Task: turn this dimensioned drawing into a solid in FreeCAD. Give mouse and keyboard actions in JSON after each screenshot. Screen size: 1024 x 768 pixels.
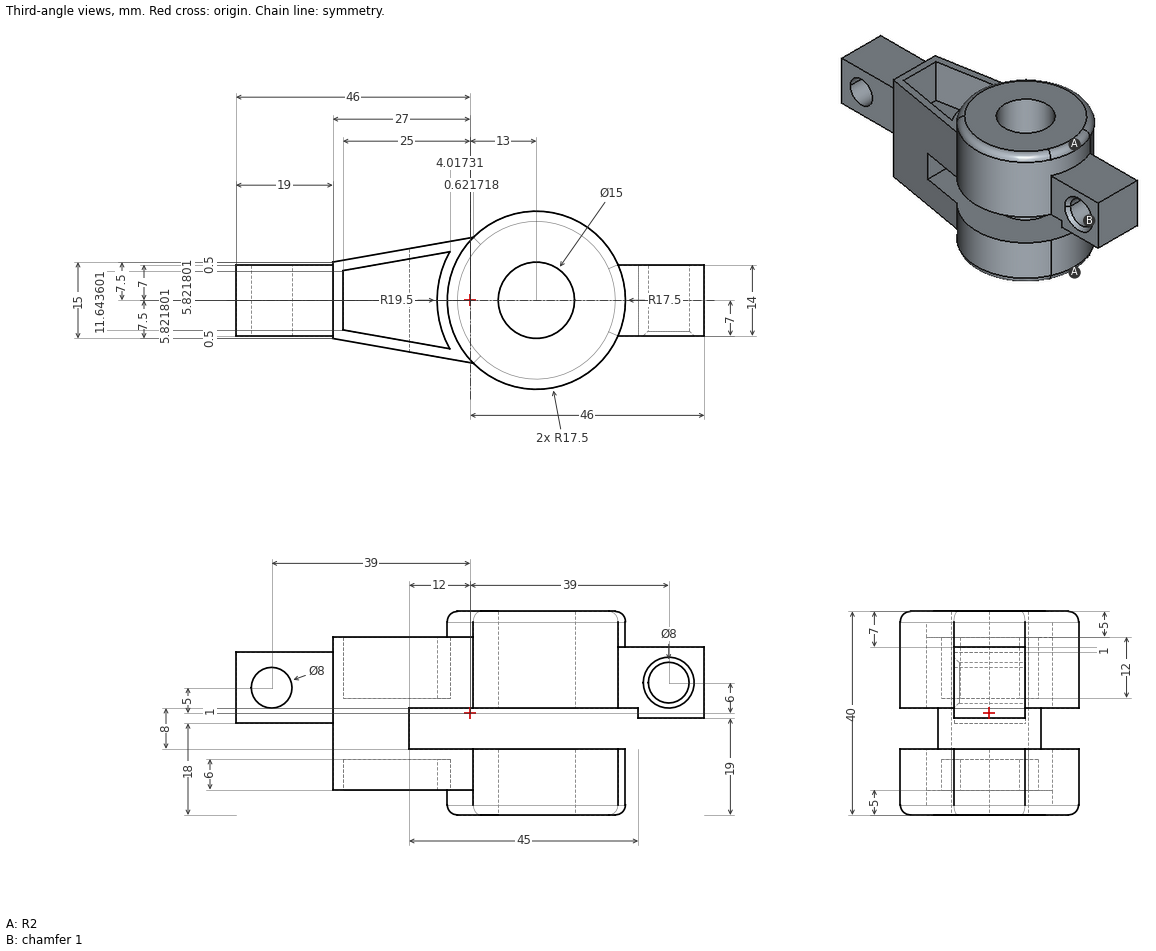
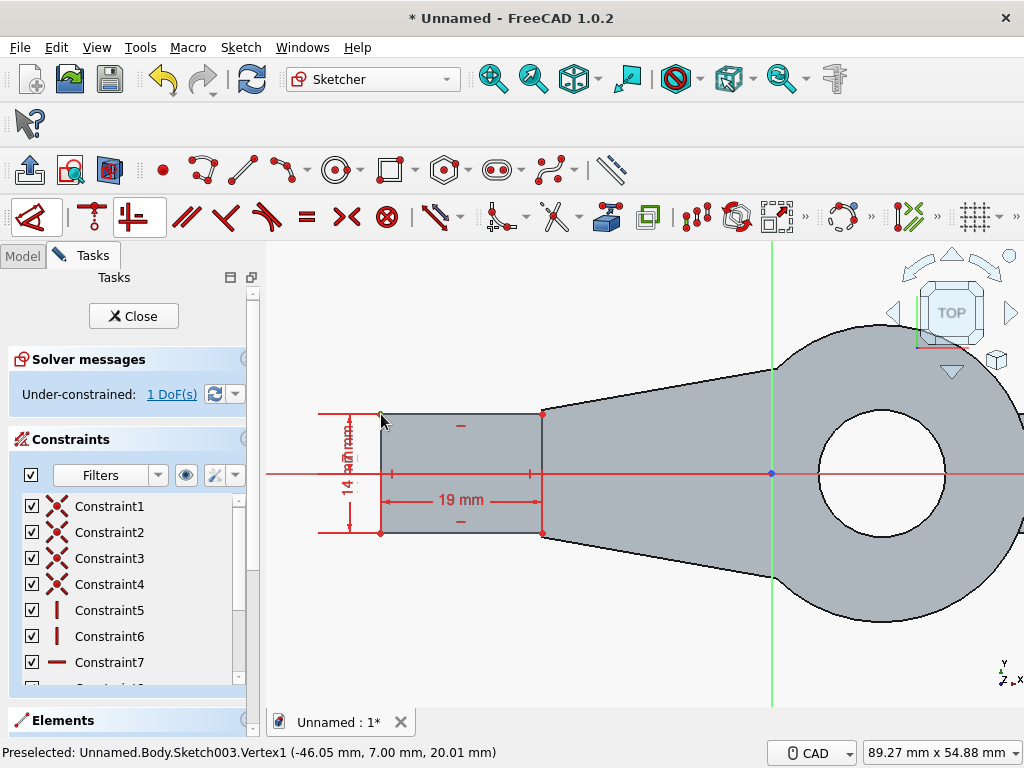
{"action": "key", "text": "l"}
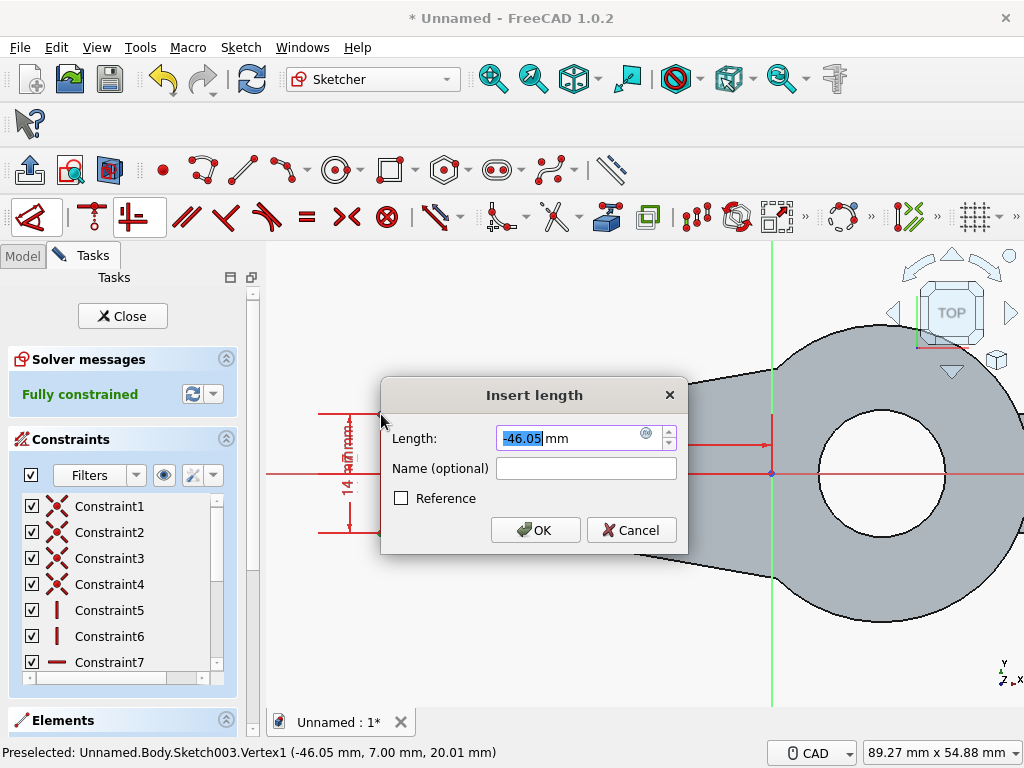
{"action": "type", "text": "-46"}
{"action": "key", "text": "Return"}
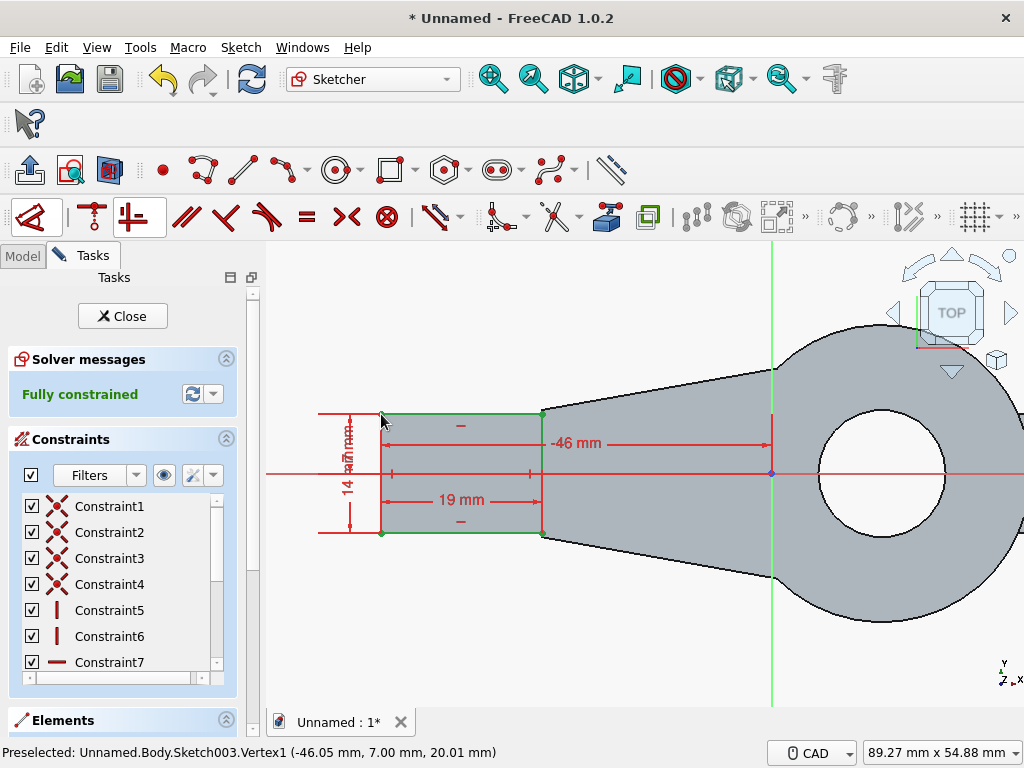
{"action": "left_click", "coordinate": [123, 316]}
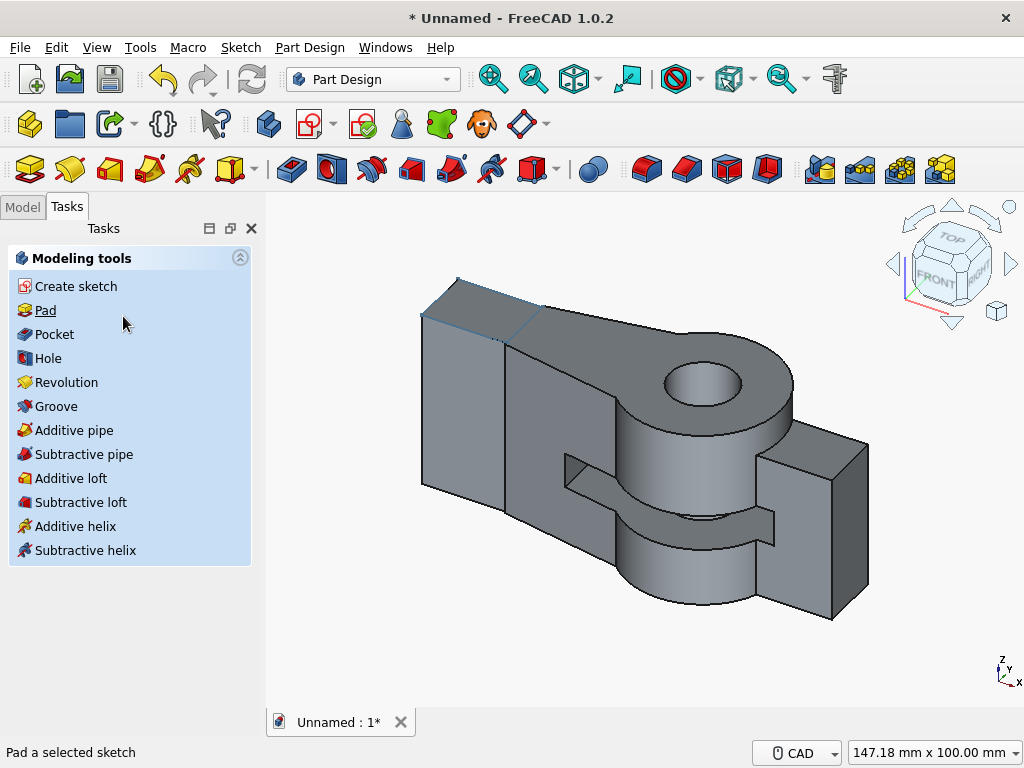
{"action": "left_click", "coordinate": [292, 170]}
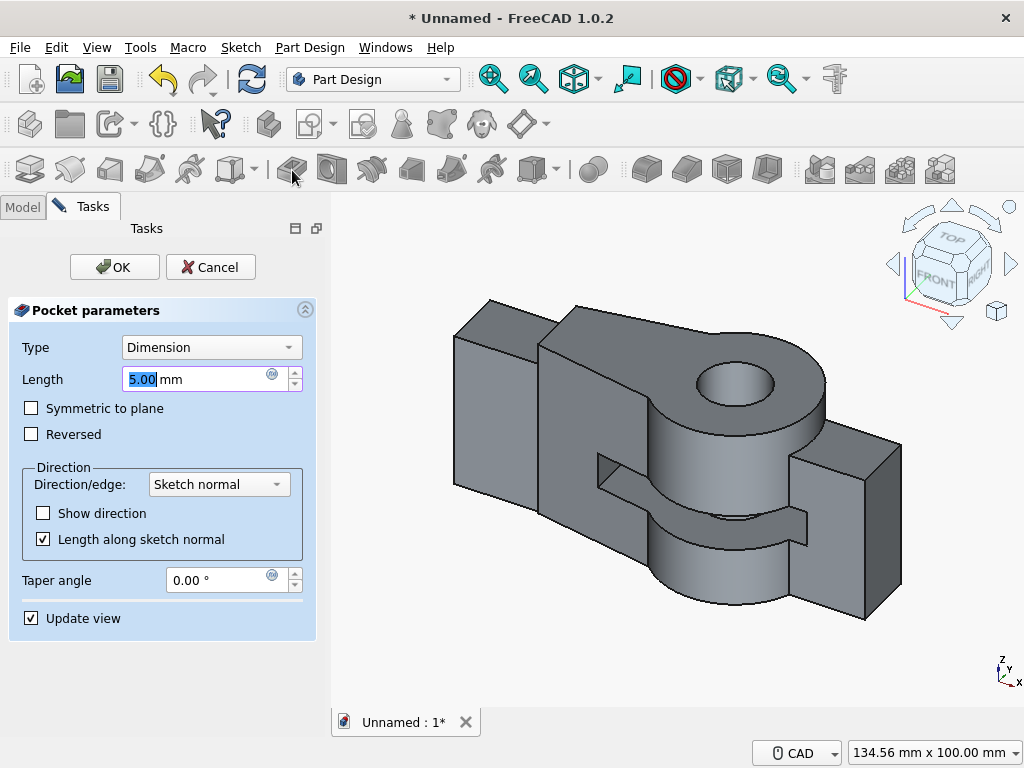
{"action": "type", "text": "7"}
{"action": "key", "text": "Tab"}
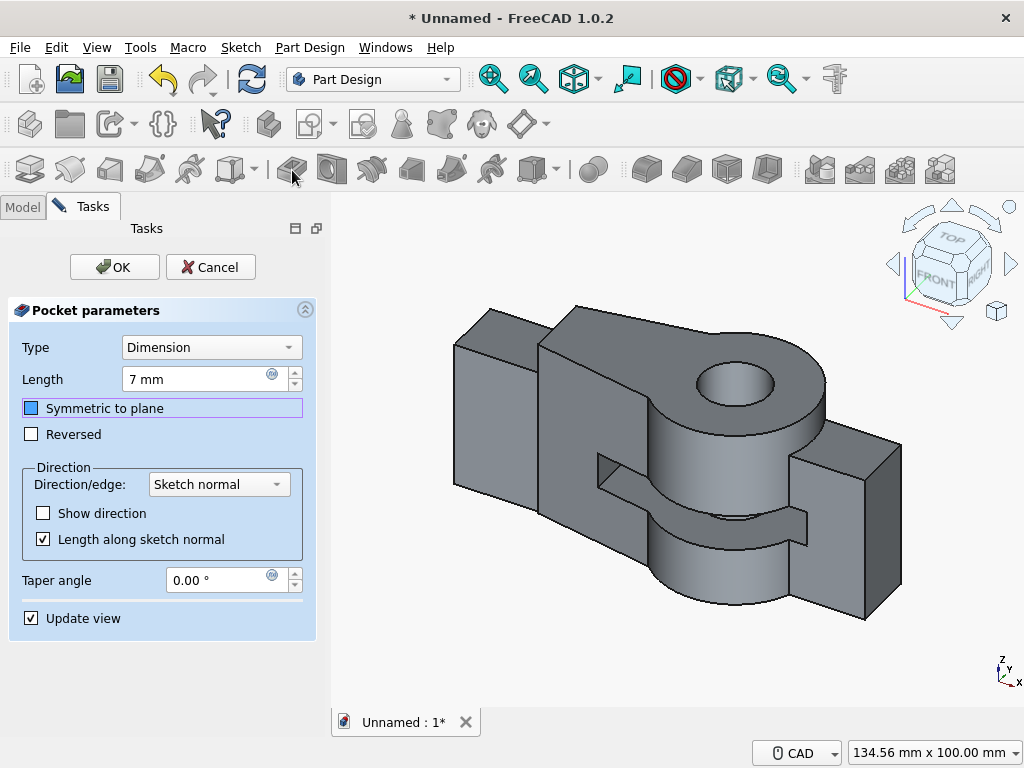
{"action": "left_click", "coordinate": [115, 267]}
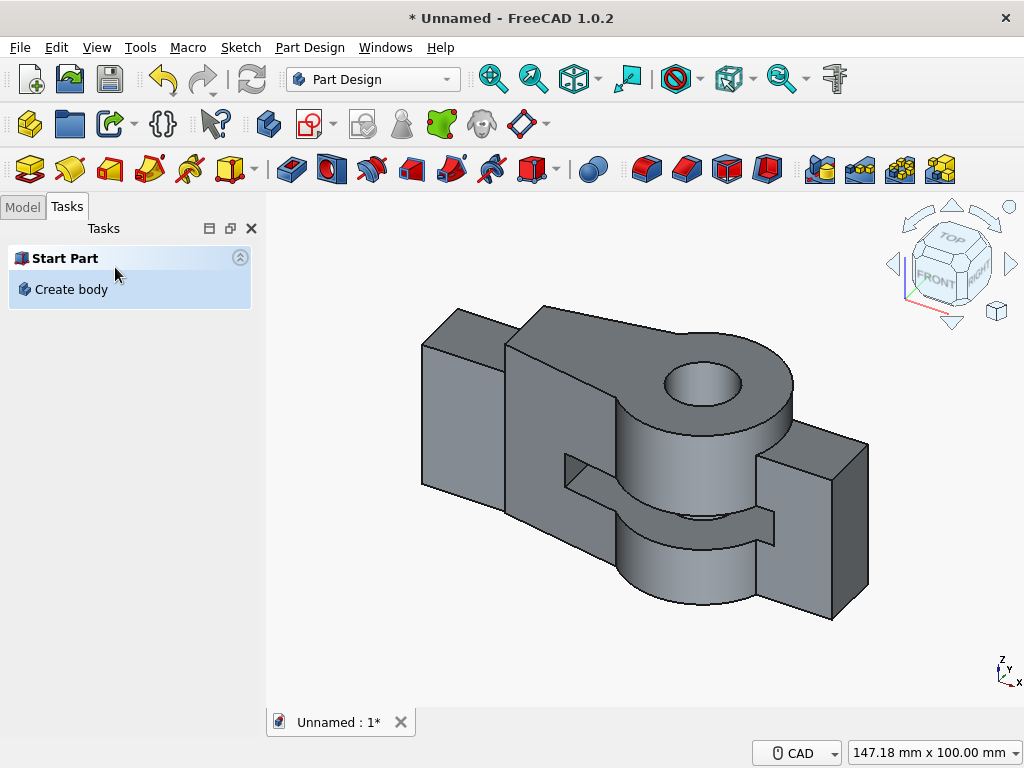
{"action": "left_click", "coordinate": [616, 355]}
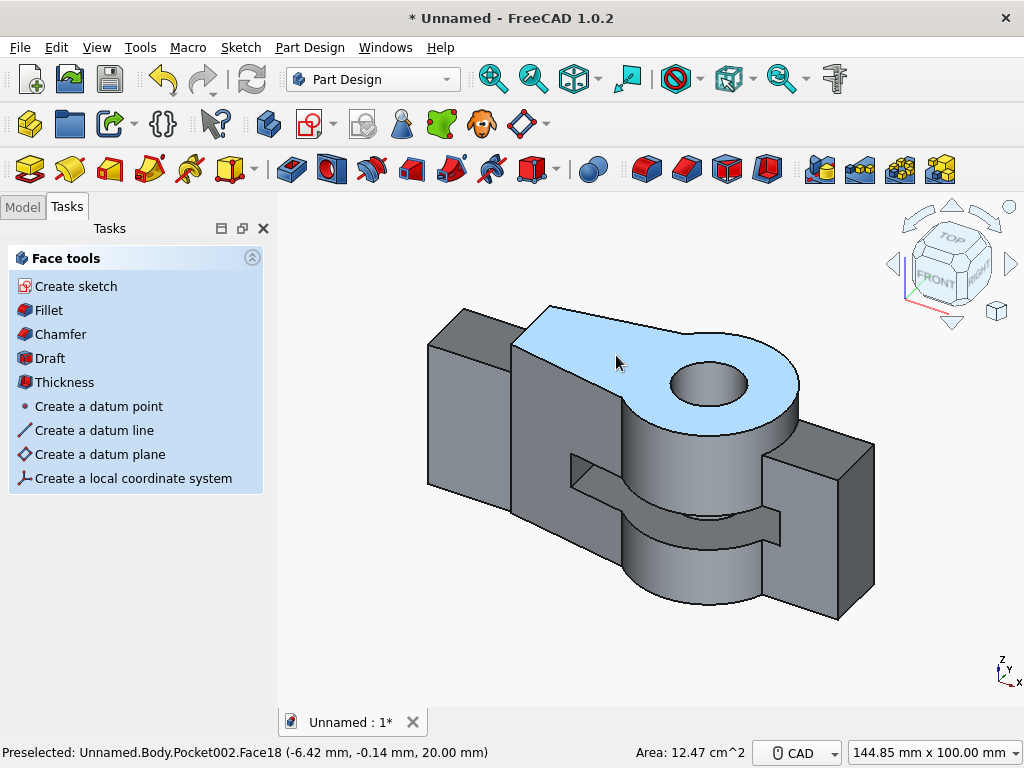
{"action": "left_click", "coordinate": [310, 124]}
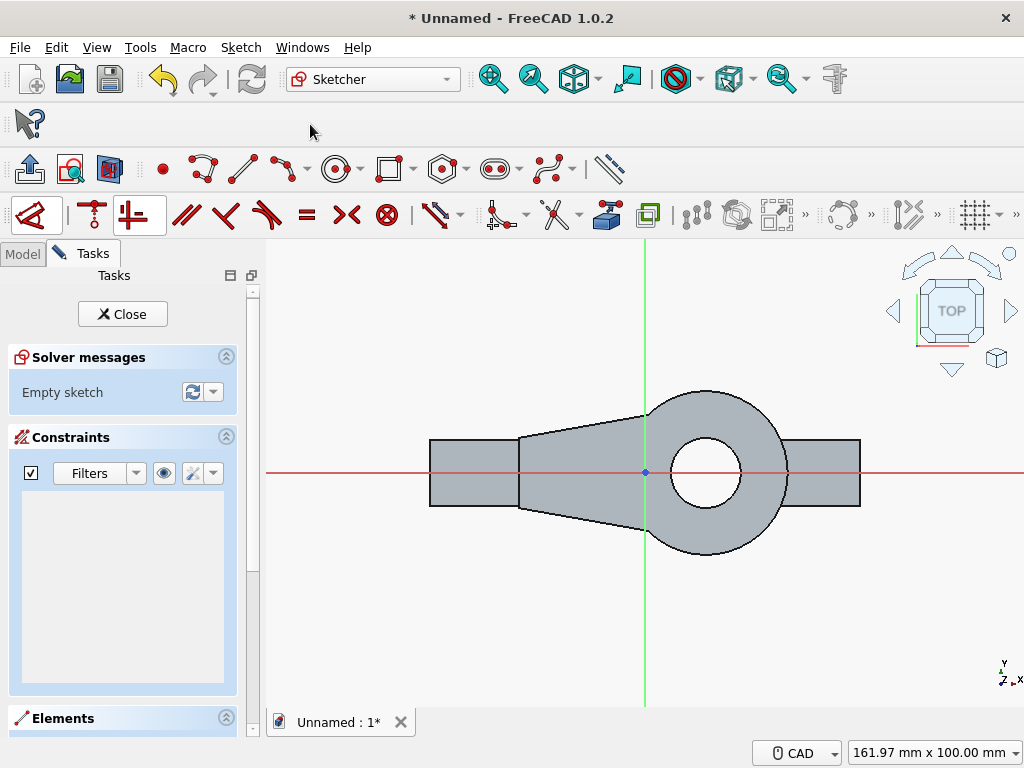
{"action": "scroll", "coordinate": [587, 473], "scroll_direction": "up", "scroll_amount": 5}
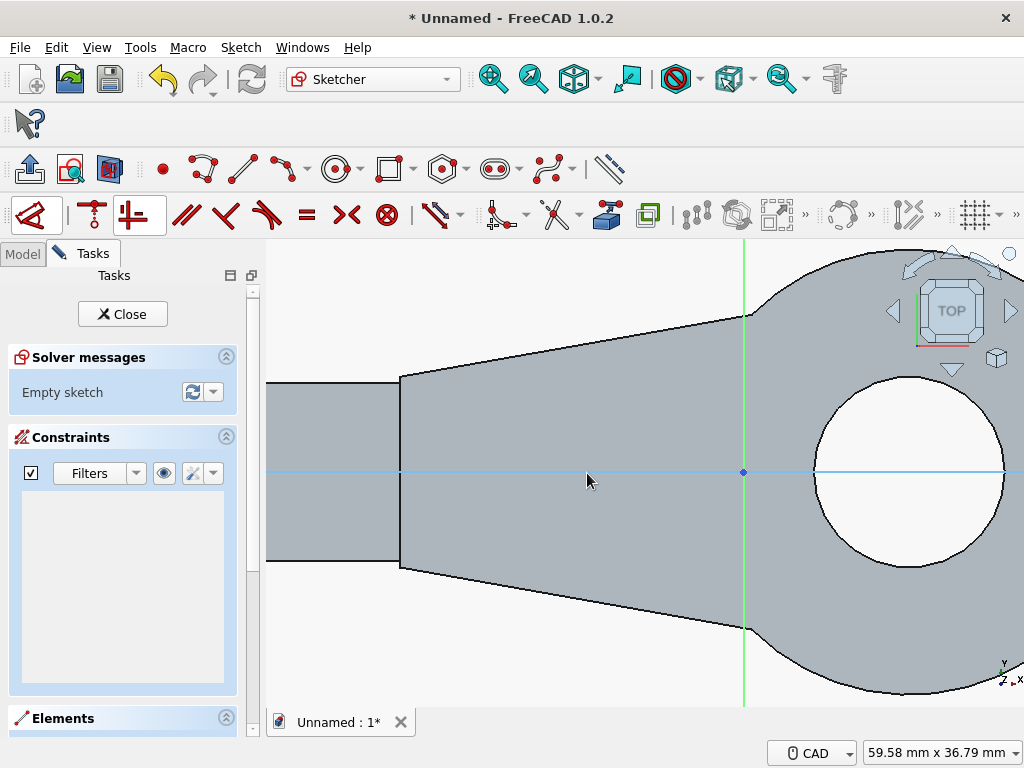
{"action": "left_click", "coordinate": [204, 170]}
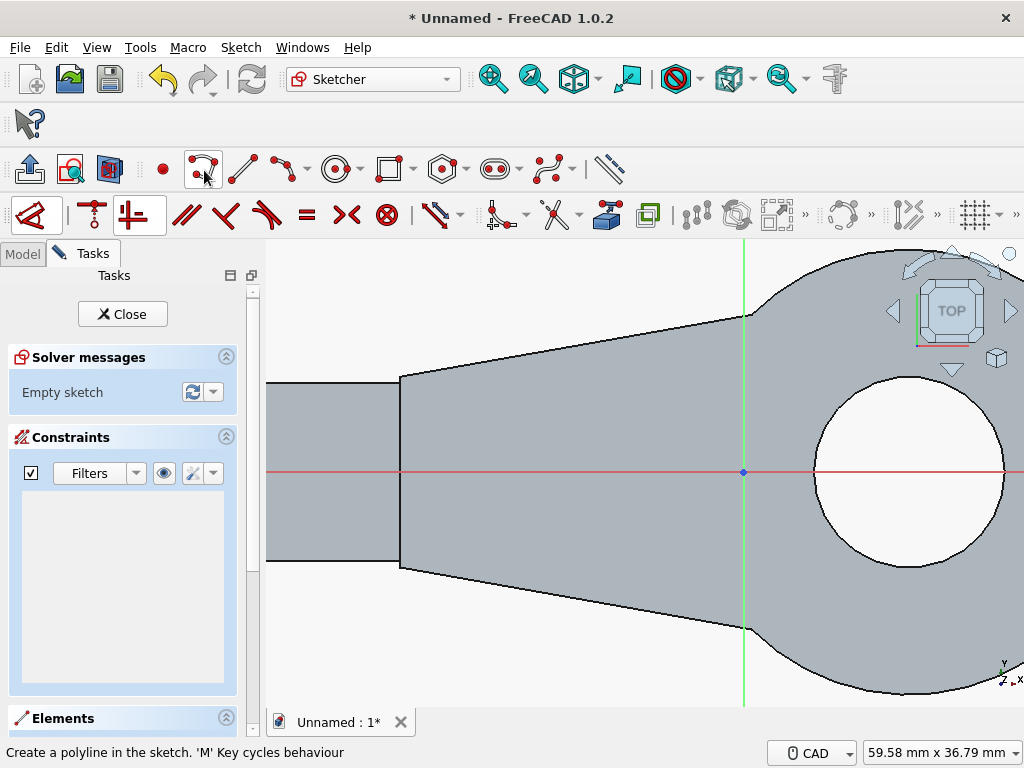
{"action": "scroll", "coordinate": [752, 315], "scroll_direction": "up", "scroll_amount": 4}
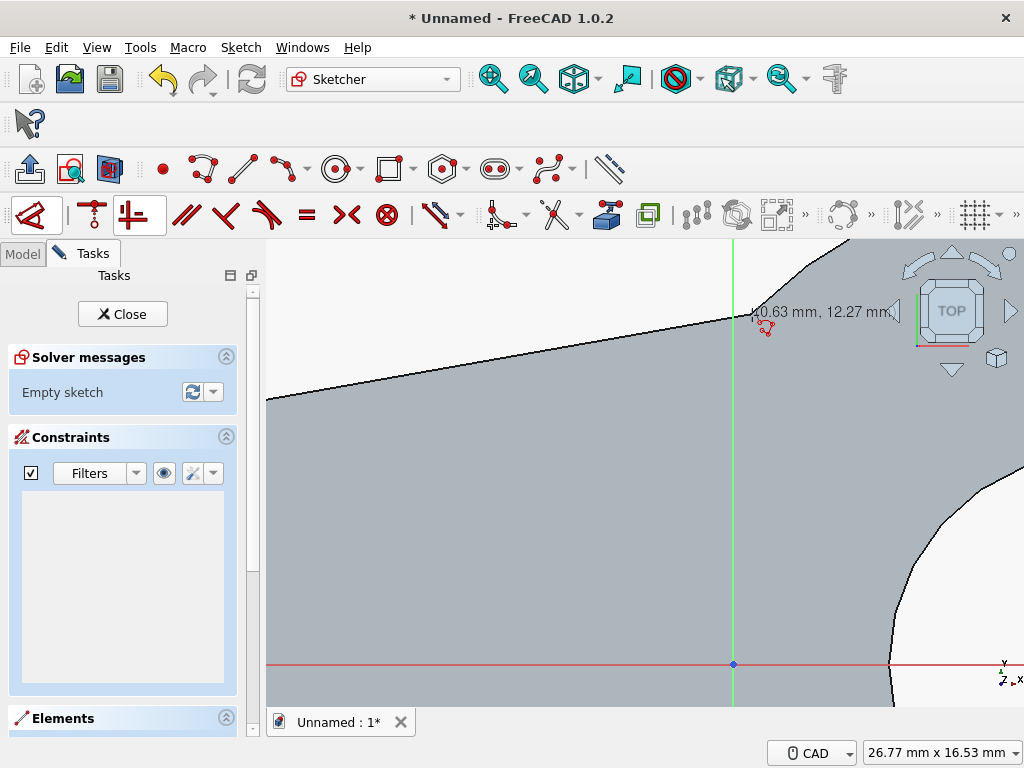
{"action": "left_click", "coordinate": [751, 314]}